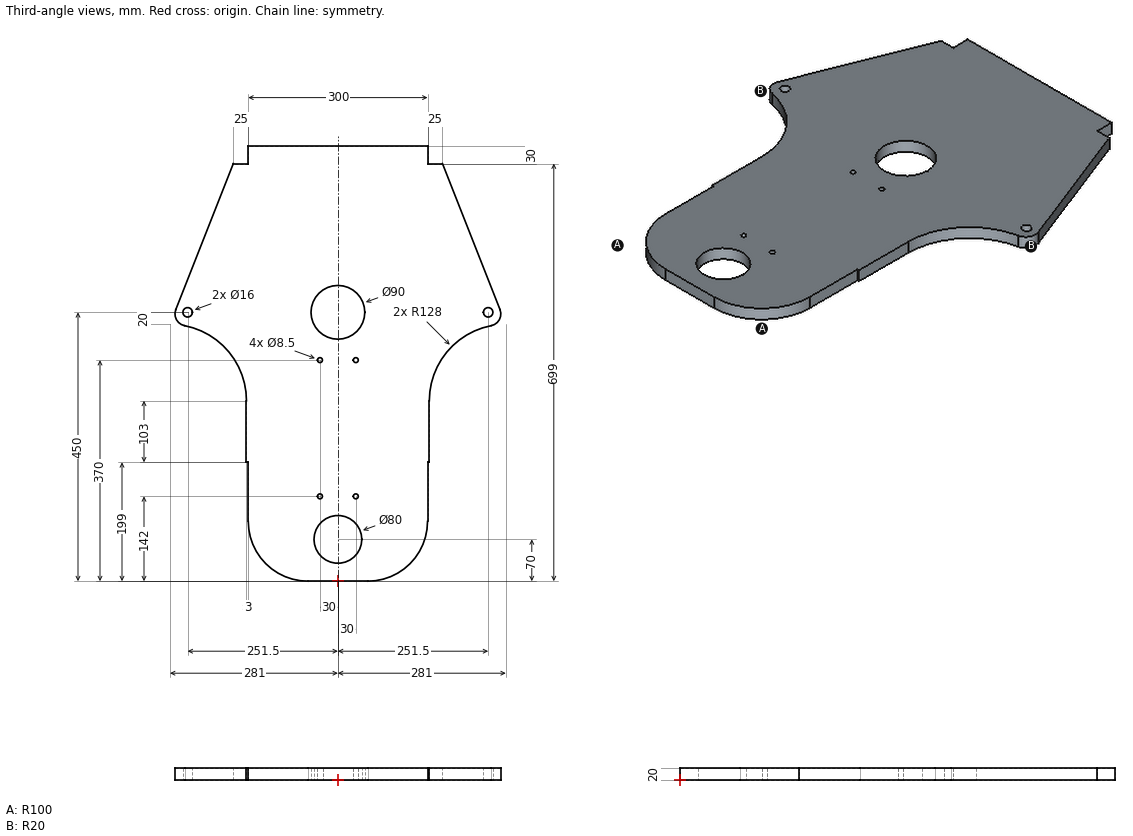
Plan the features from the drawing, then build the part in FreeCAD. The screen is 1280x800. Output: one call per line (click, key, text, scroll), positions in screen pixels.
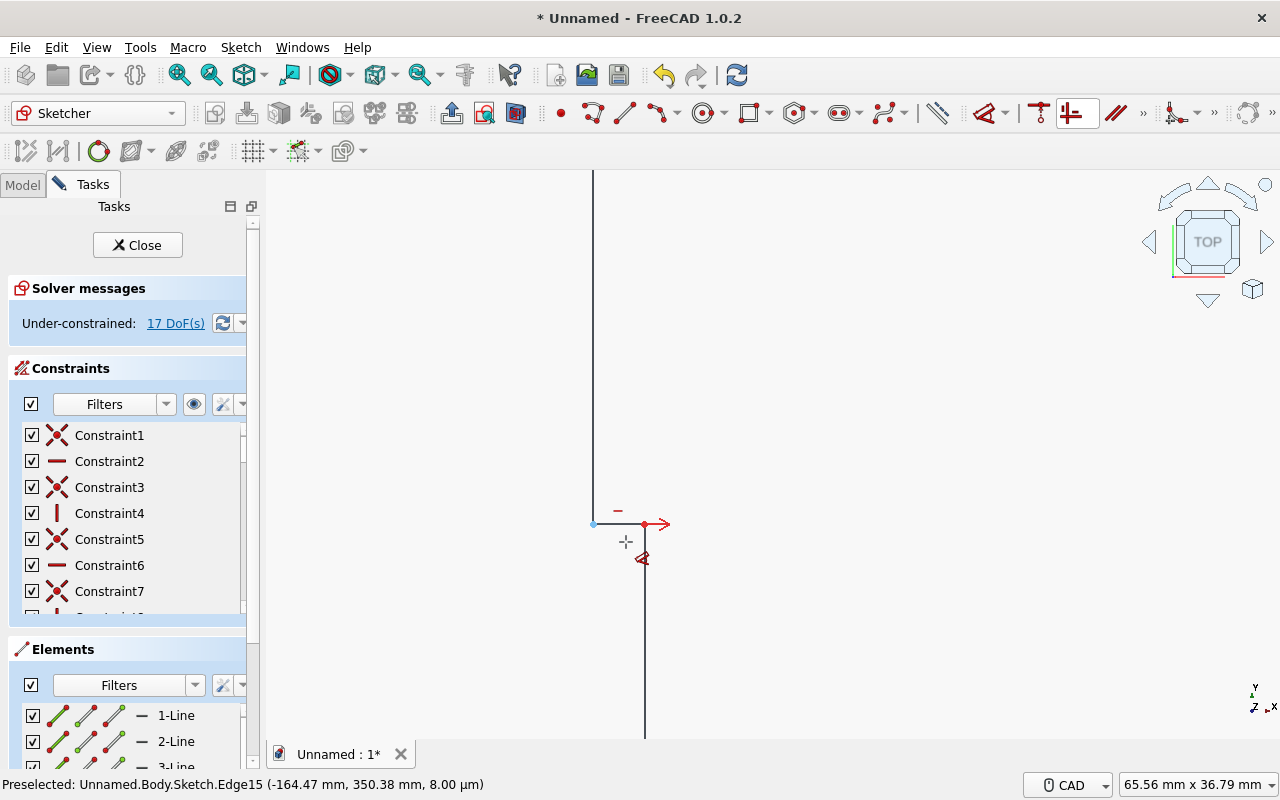
click(619, 524)
click(619, 558)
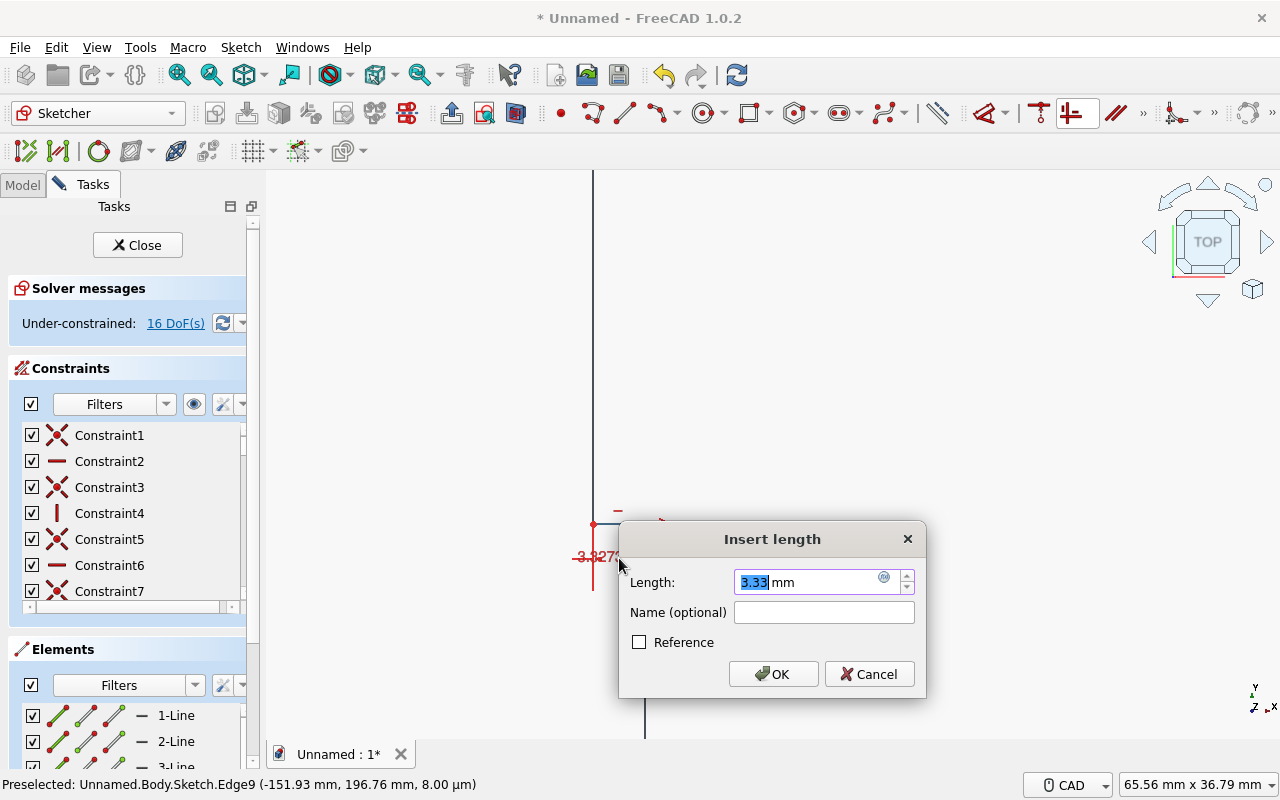
text(3)
key(Return)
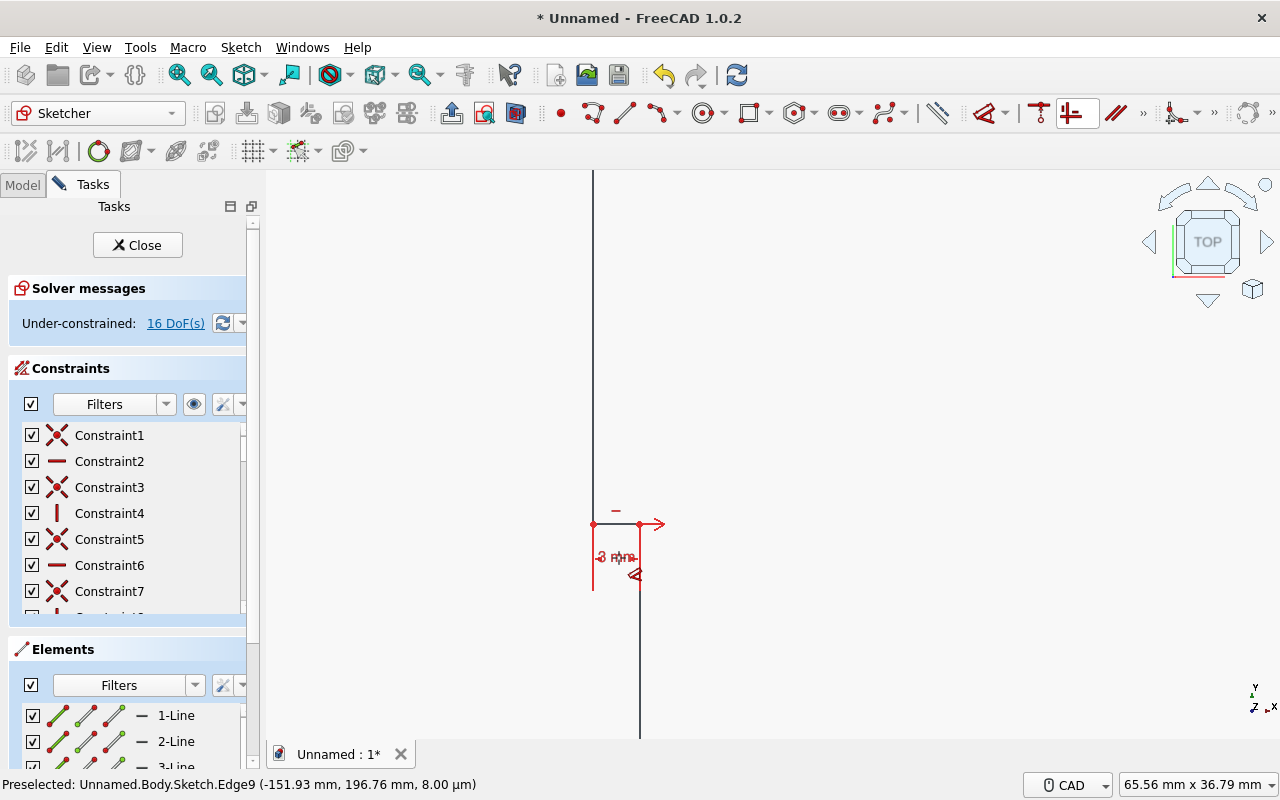
scroll(608, 562, down, 16)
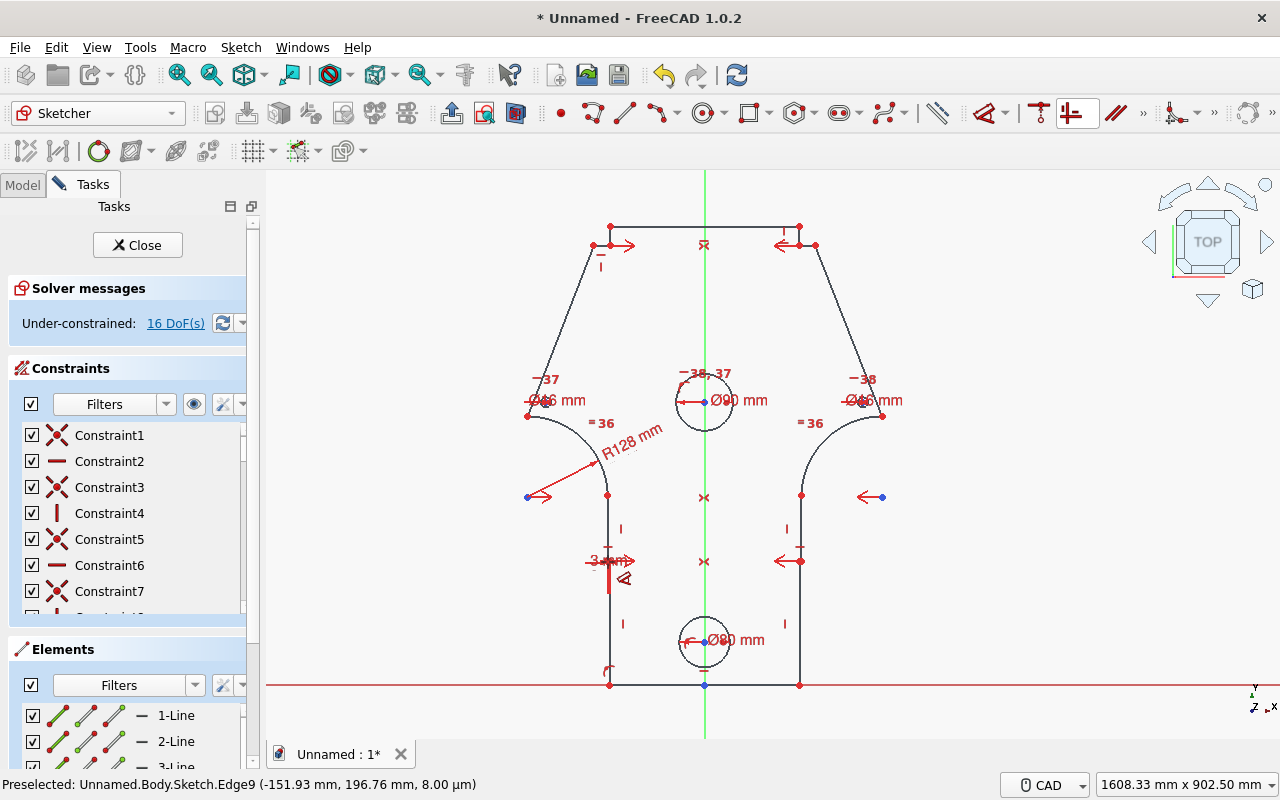
scroll(810, 246, up, 6)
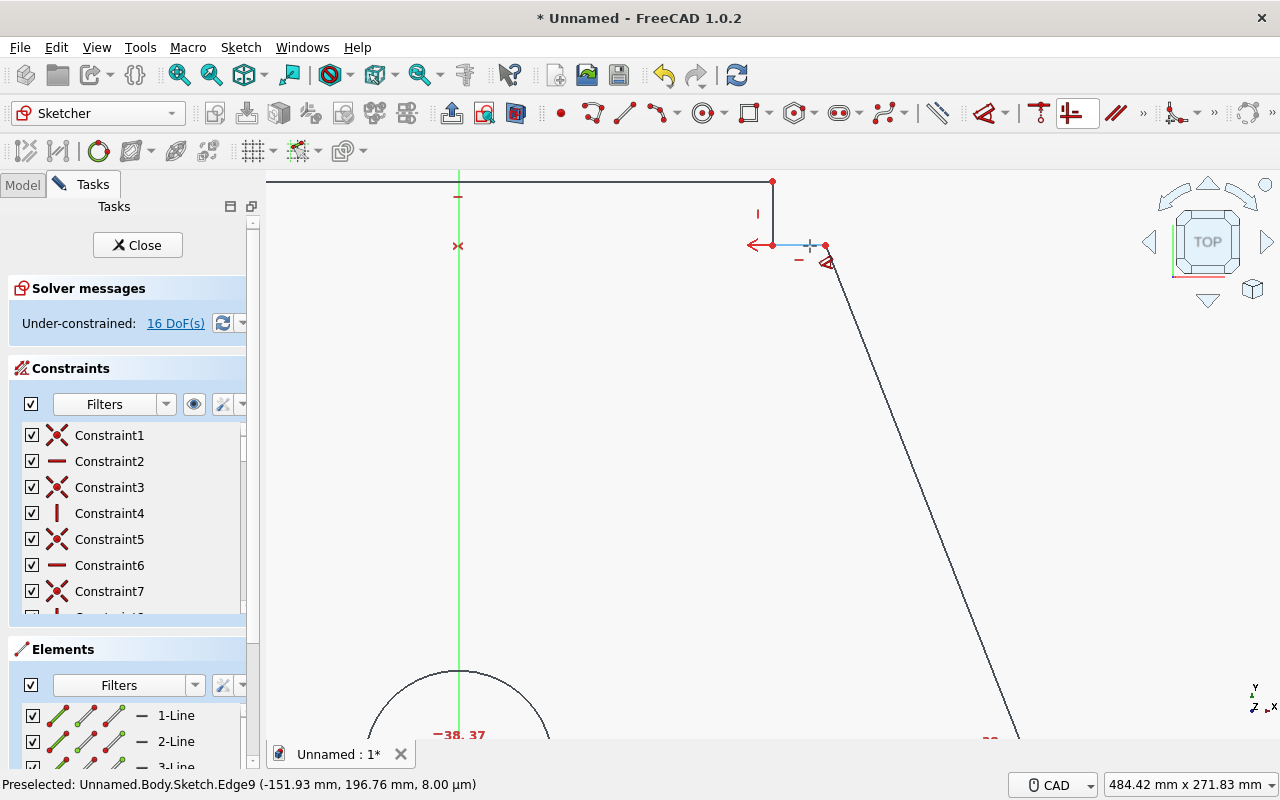
click(810, 245)
click(799, 211)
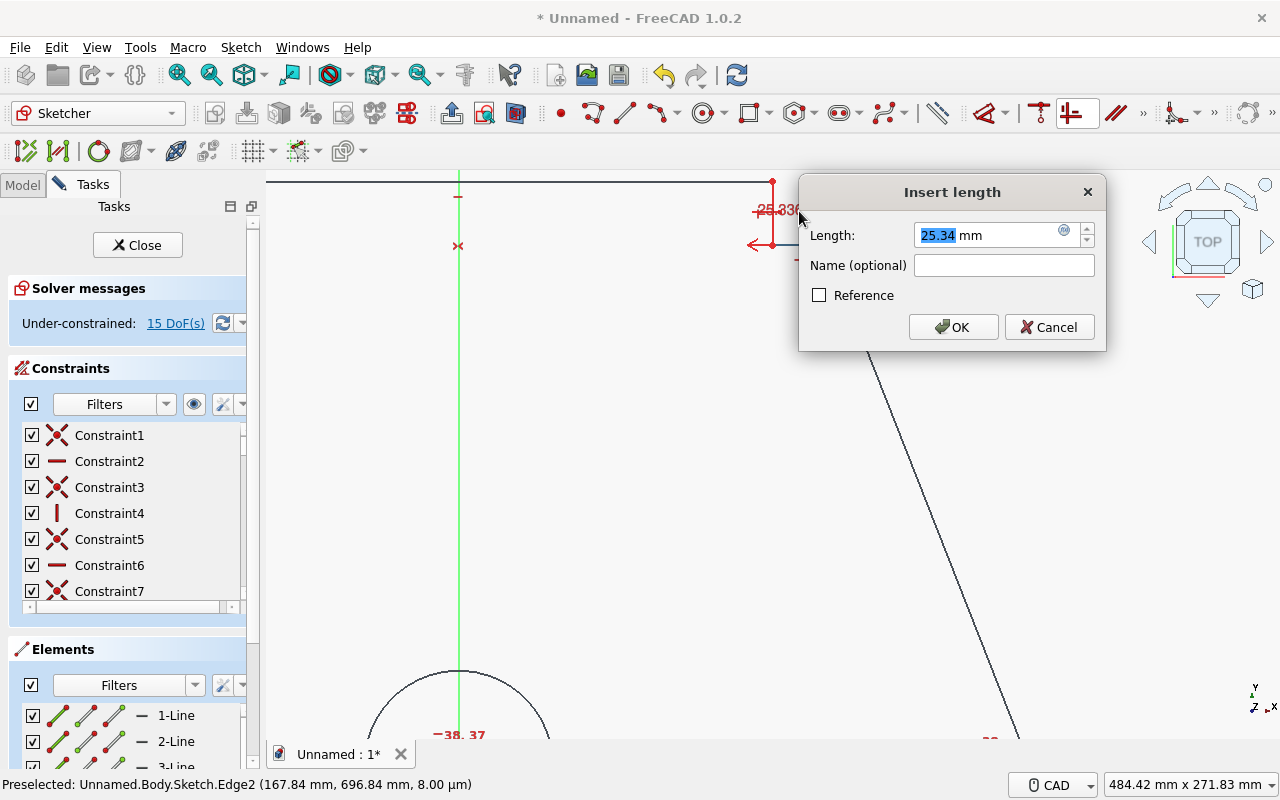
text(25)
key(Return)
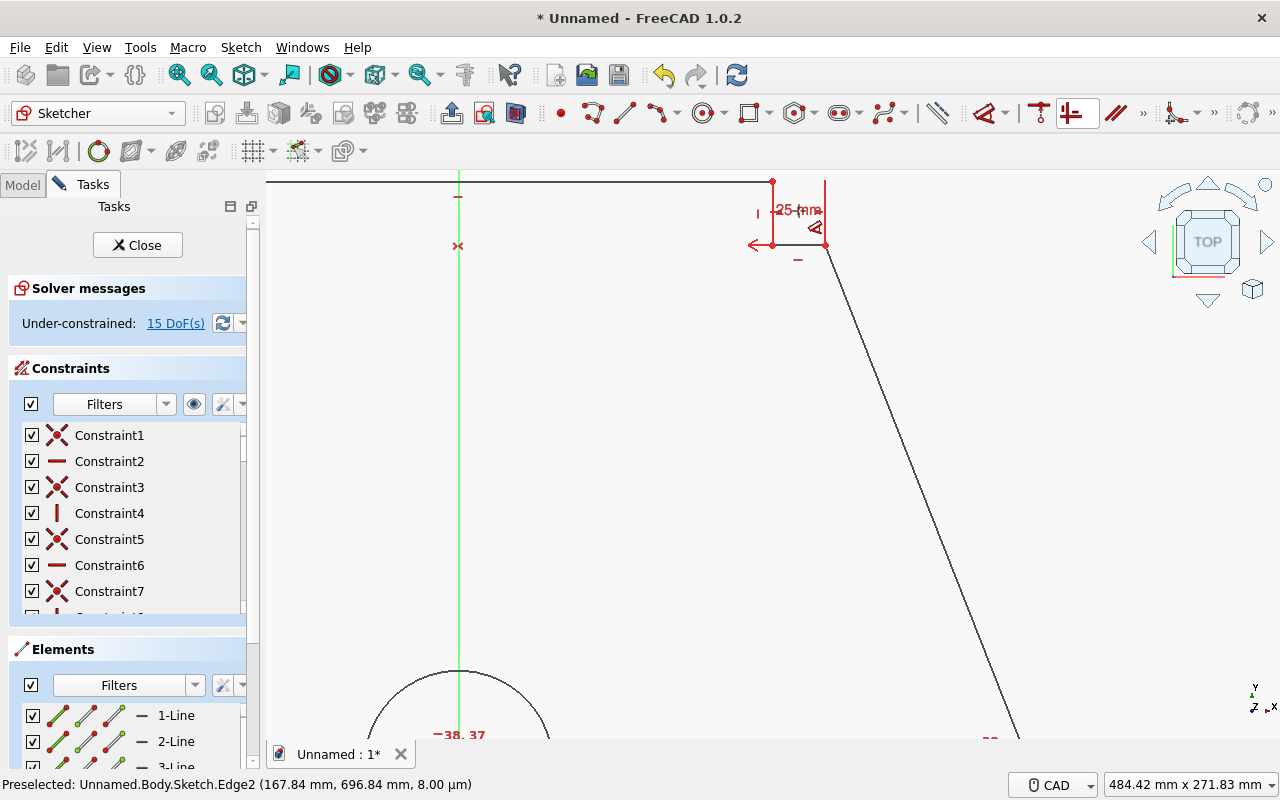
click(773, 226)
click(739, 232)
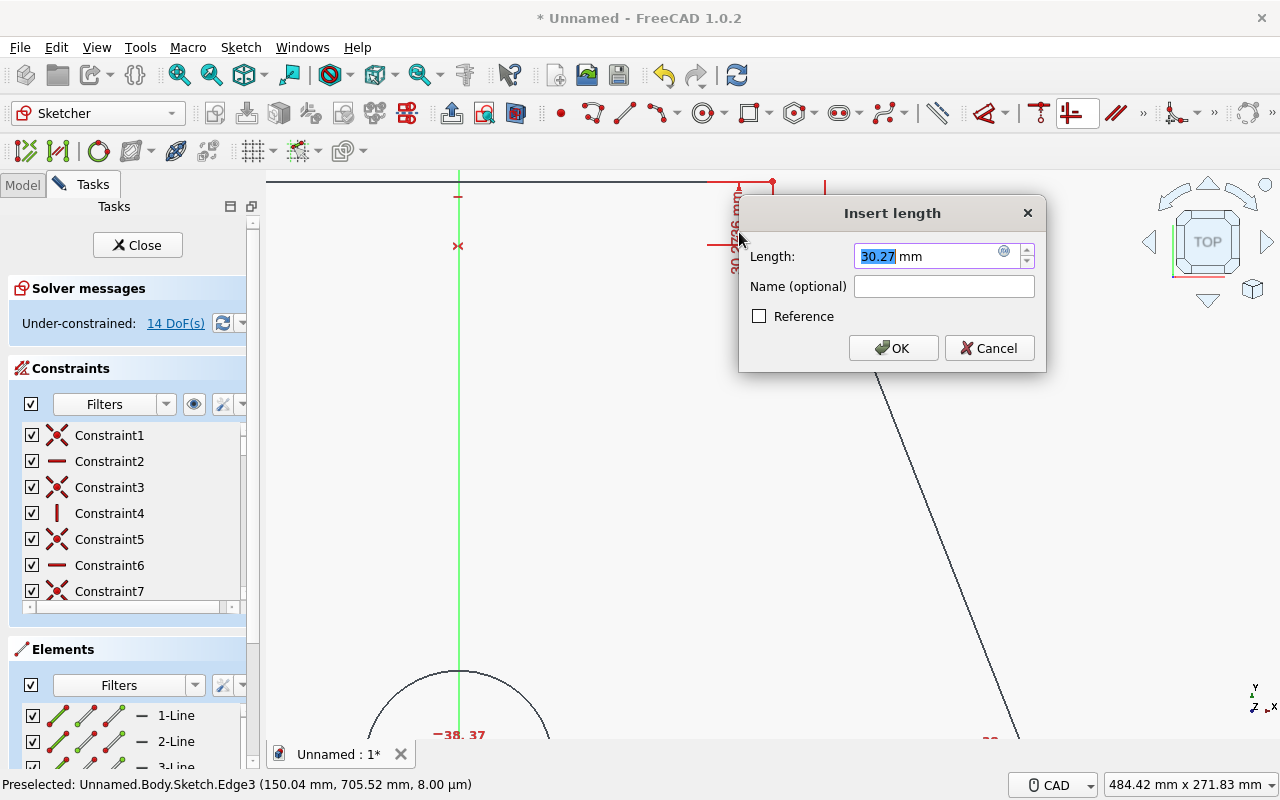
text(30)
key(Return)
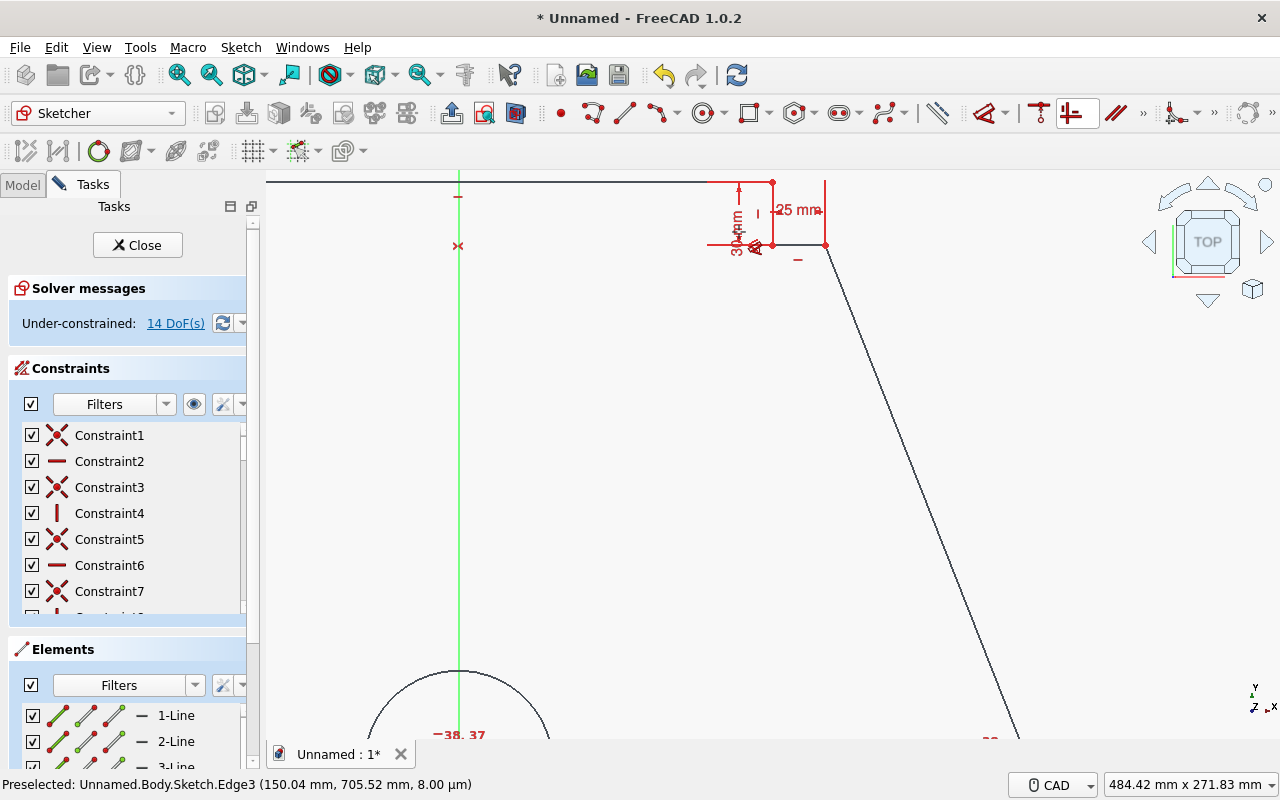
scroll(785, 295, down, 7)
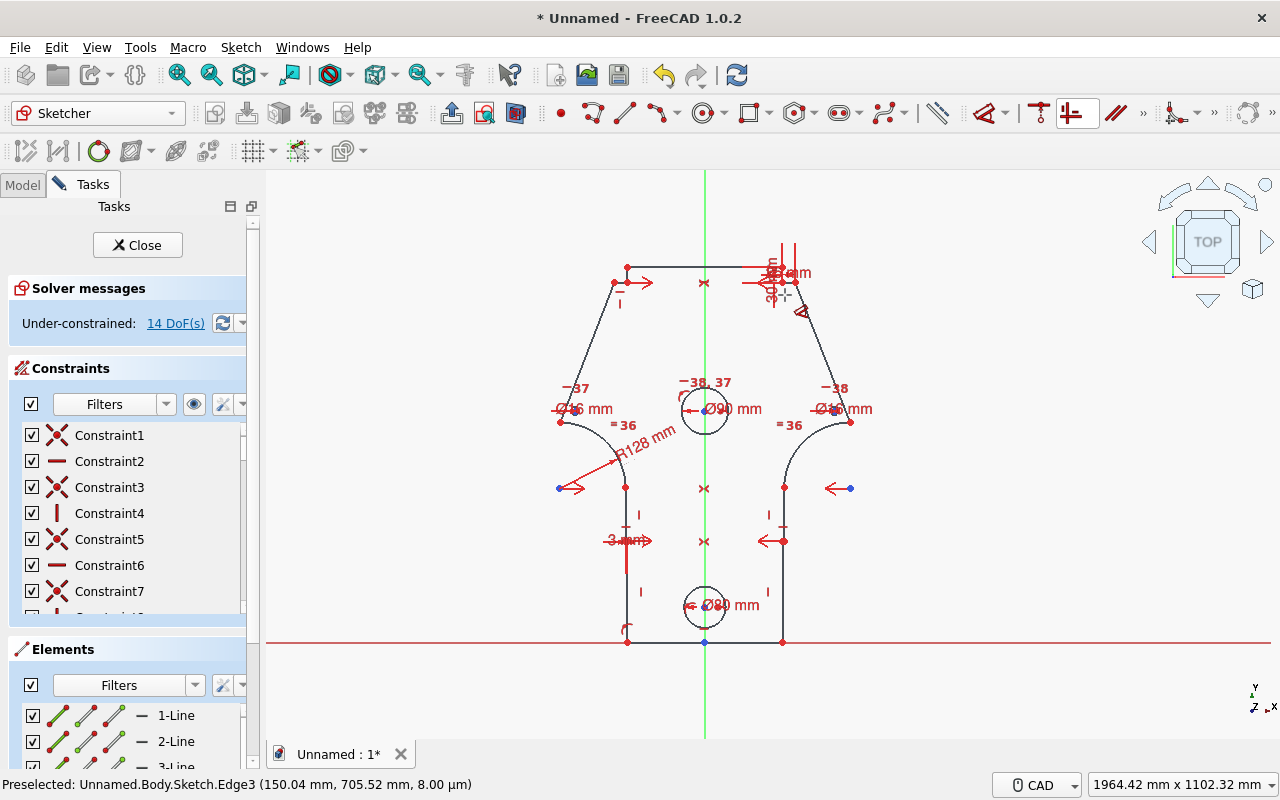
scroll(624, 283, up, 7)